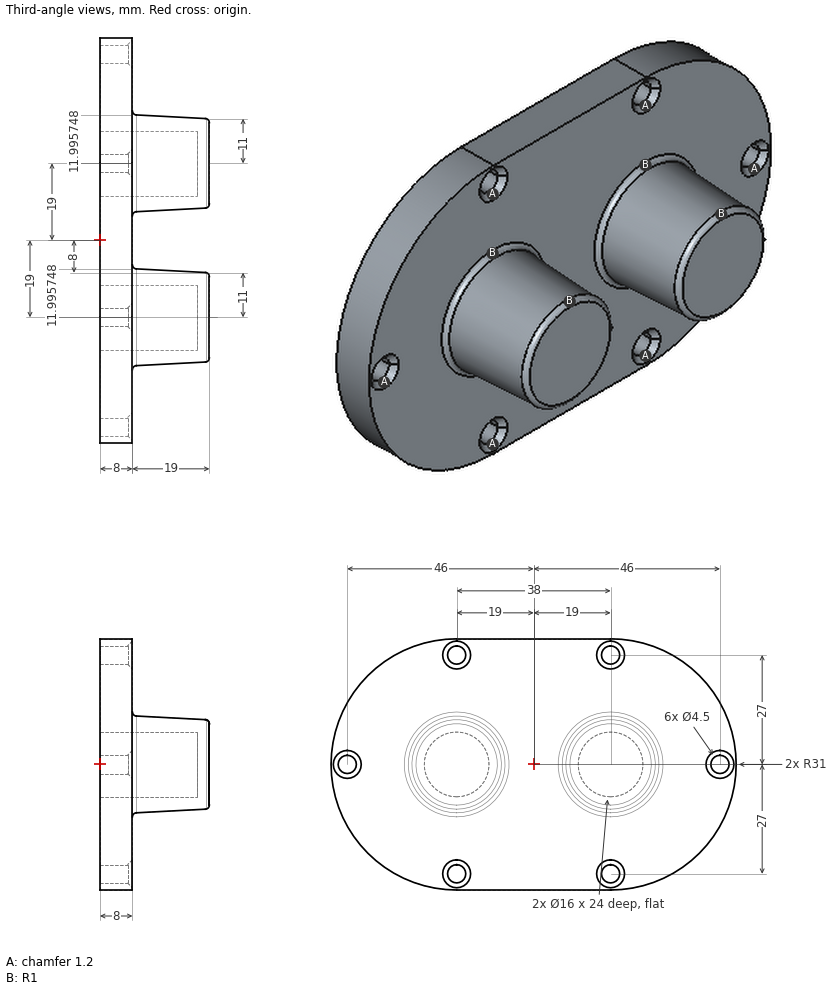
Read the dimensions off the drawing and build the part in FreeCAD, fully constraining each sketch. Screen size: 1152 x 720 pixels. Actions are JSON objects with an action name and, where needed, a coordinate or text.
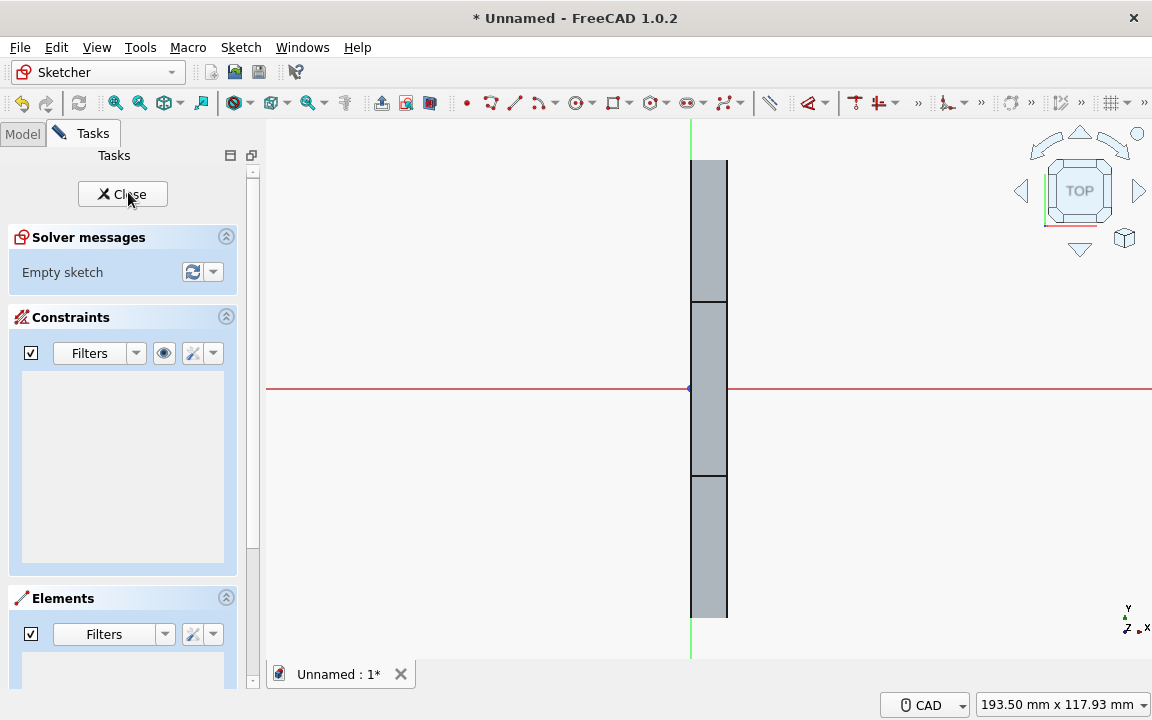
{"action": "left_click", "coordinate": [430, 104]}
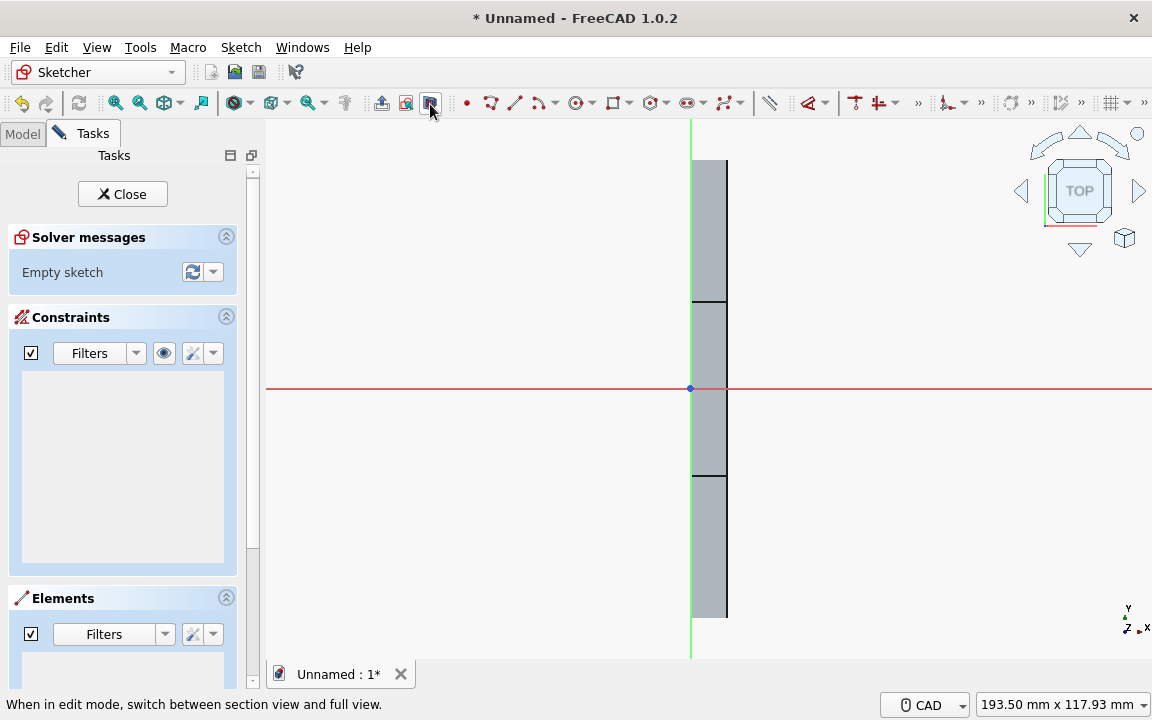
{"action": "scroll", "coordinate": [826, 451], "scroll_direction": "up", "scroll_amount": 6}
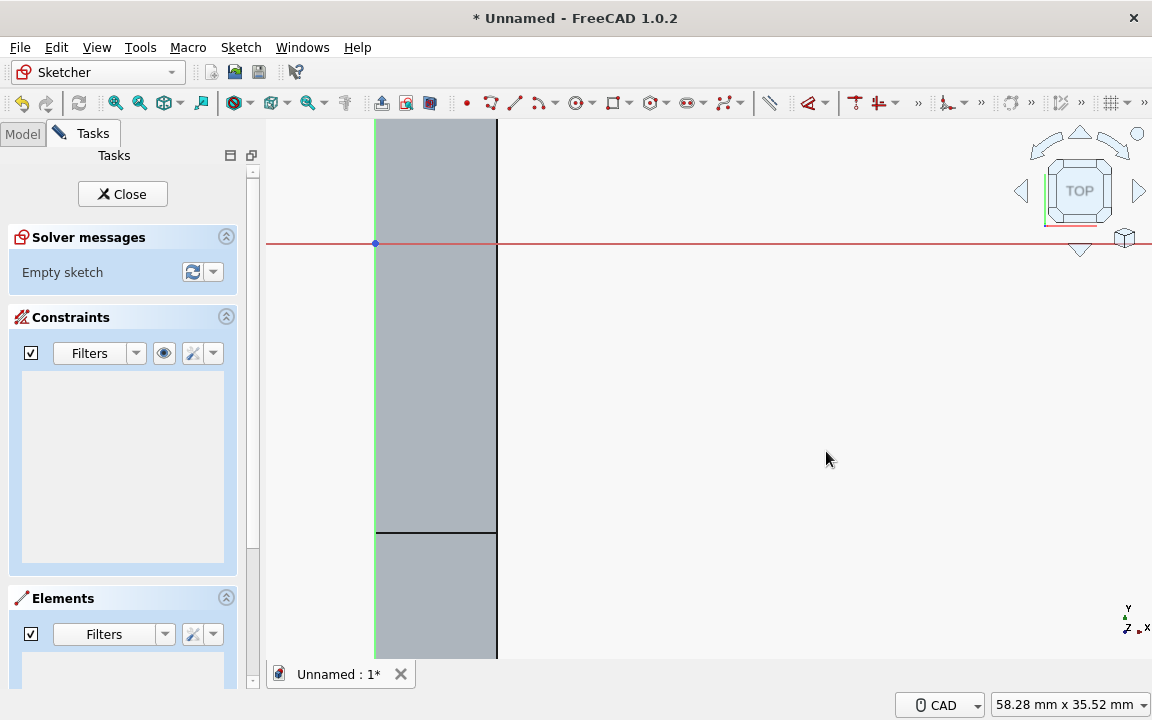
{"action": "left_click", "coordinate": [492, 104]}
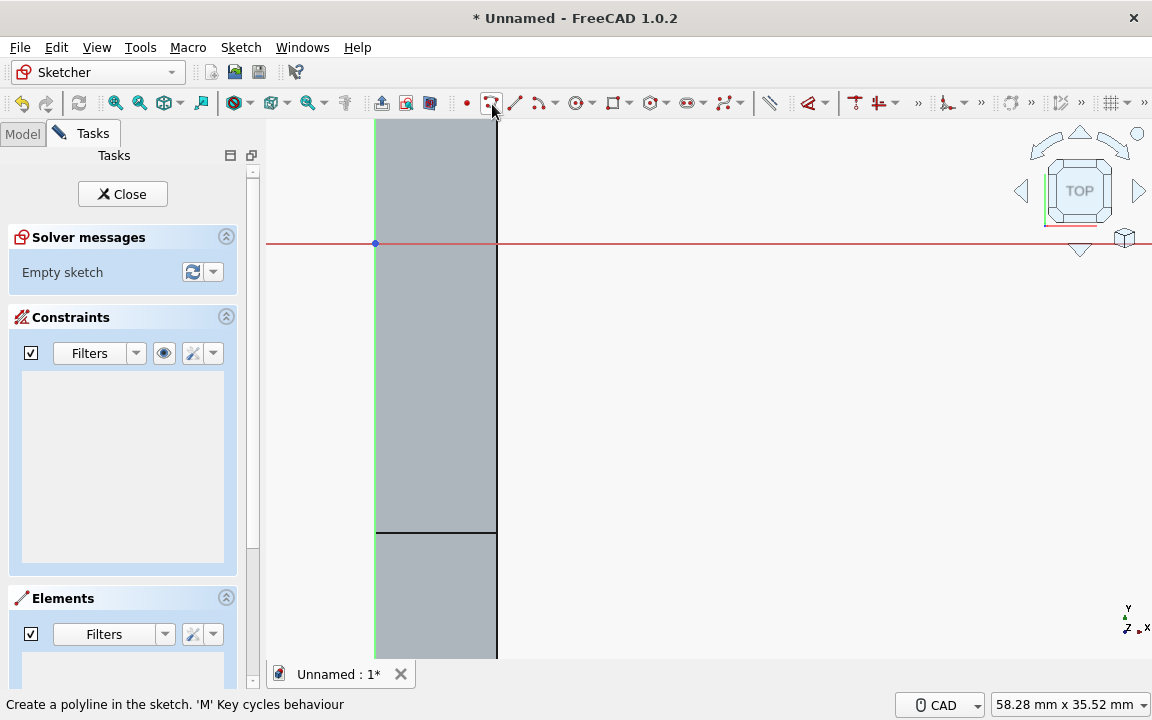
{"action": "left_click", "coordinate": [497, 350]}
{"action": "left_click", "coordinate": [497, 533]}
{"action": "left_click", "coordinate": [786, 533]}
{"action": "left_click", "coordinate": [786, 365]}
{"action": "left_click", "coordinate": [497, 351]}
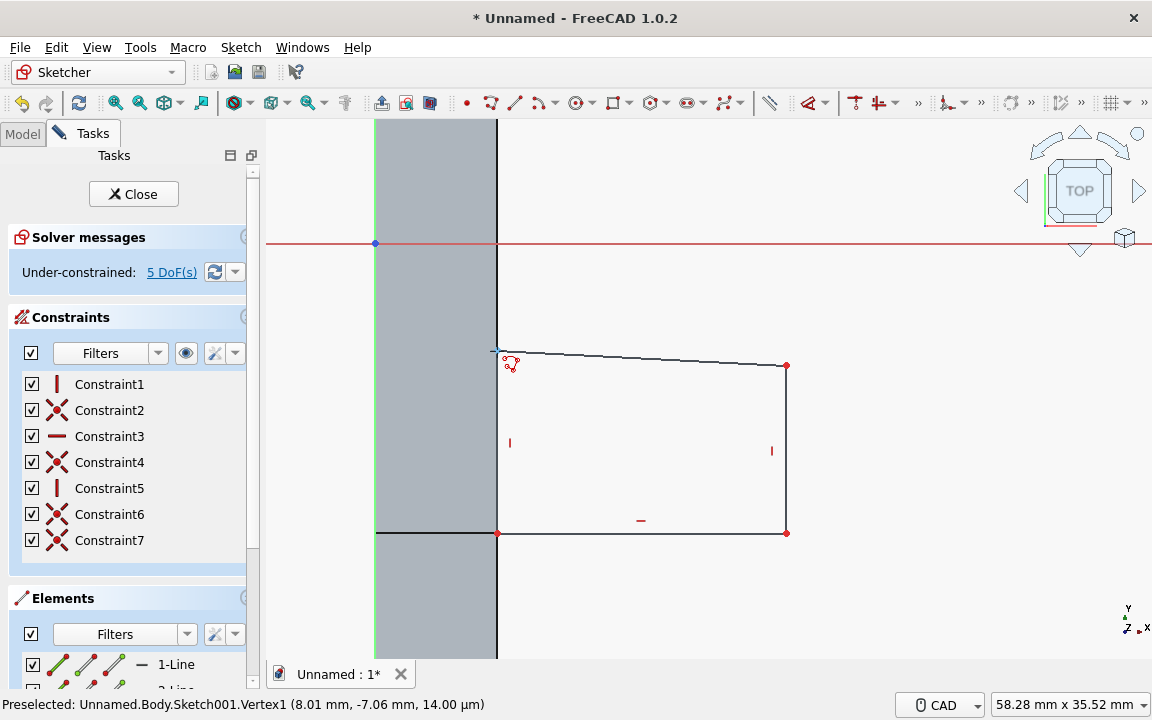
{"action": "left_click", "coordinate": [516, 104]}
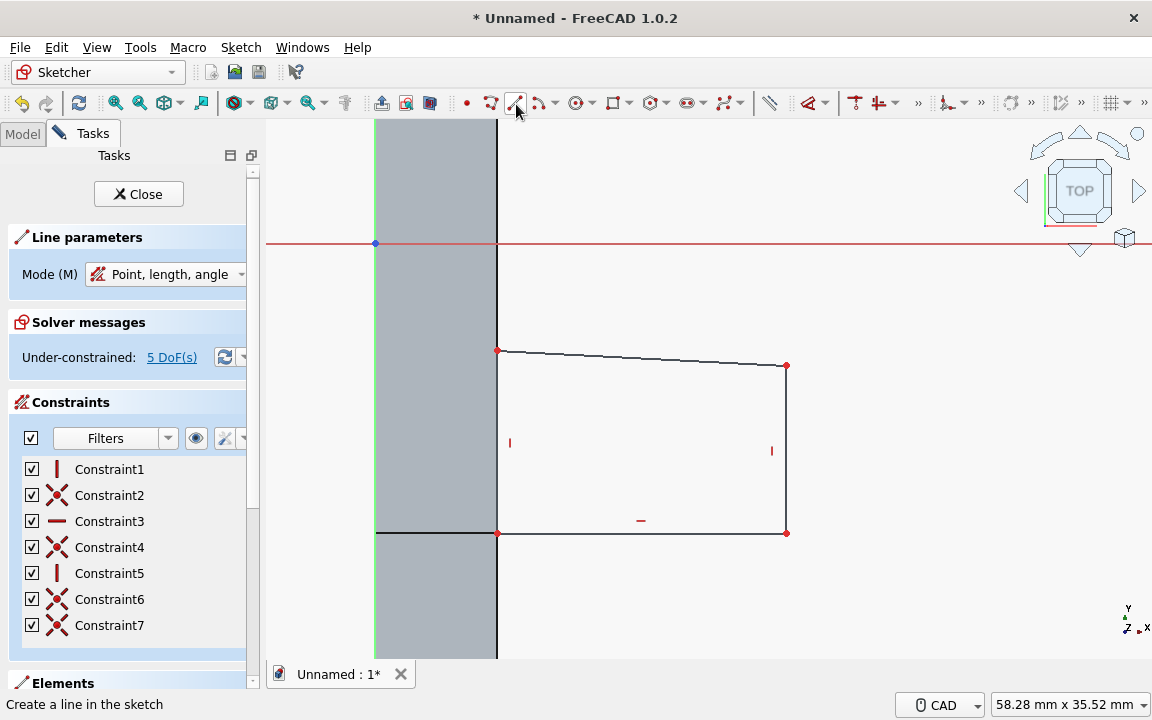
{"action": "left_click", "coordinate": [815, 533]}
{"action": "left_click", "coordinate": [901, 533]}
{"action": "key", "text": "Escape"}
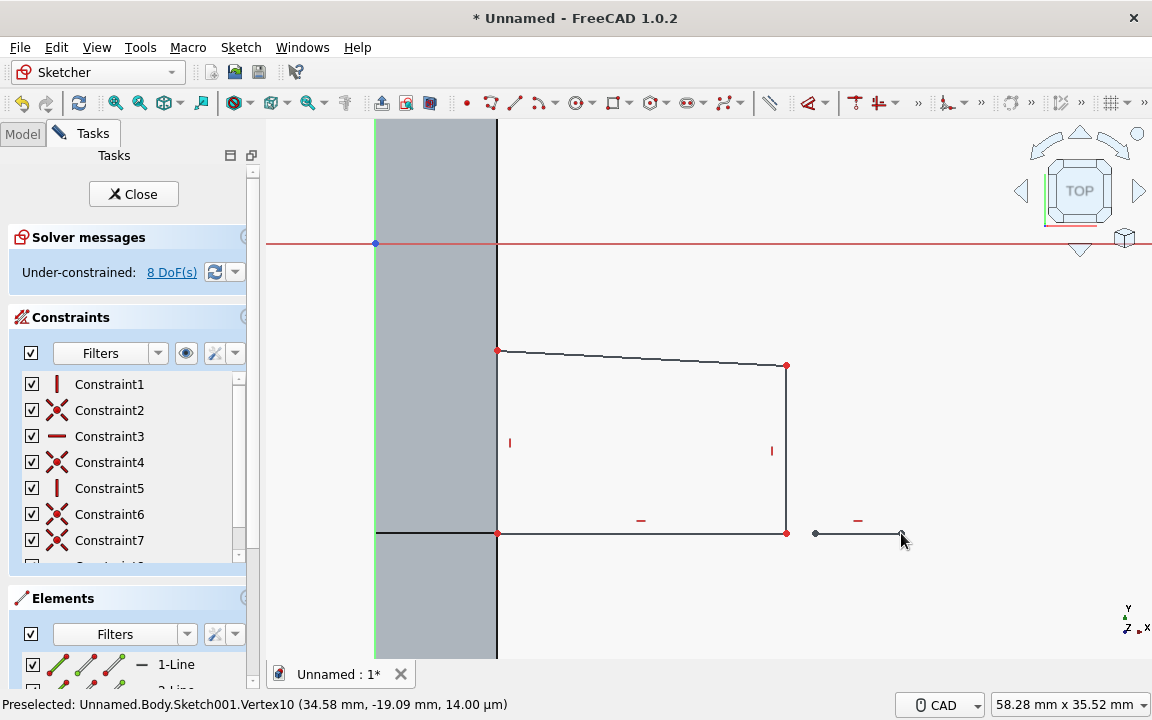
{"action": "left_click", "coordinate": [841, 534]}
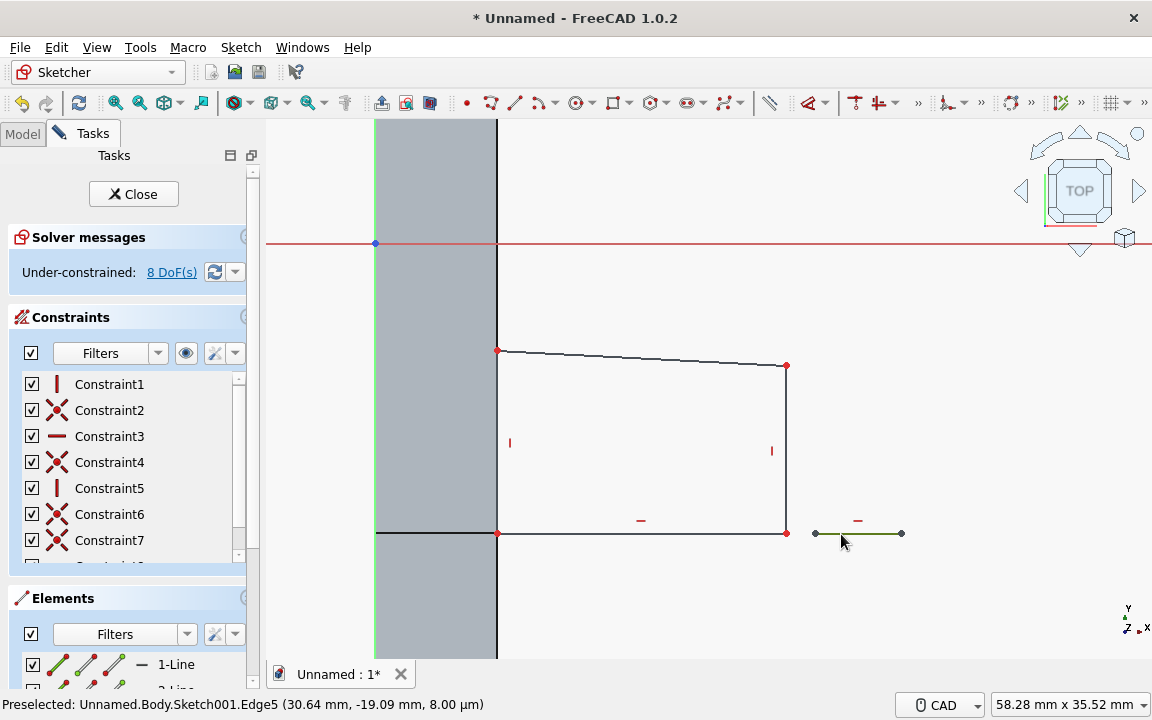
{"action": "left_click", "coordinate": [770, 104]}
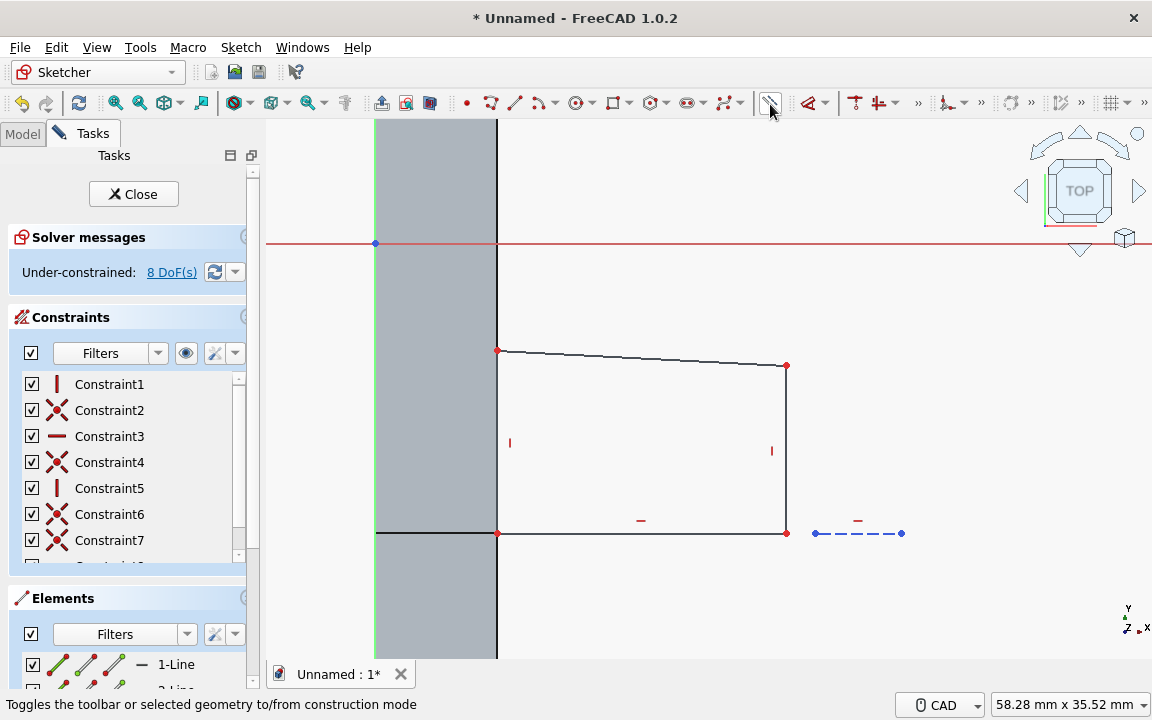
{"action": "left_click", "coordinate": [808, 104]}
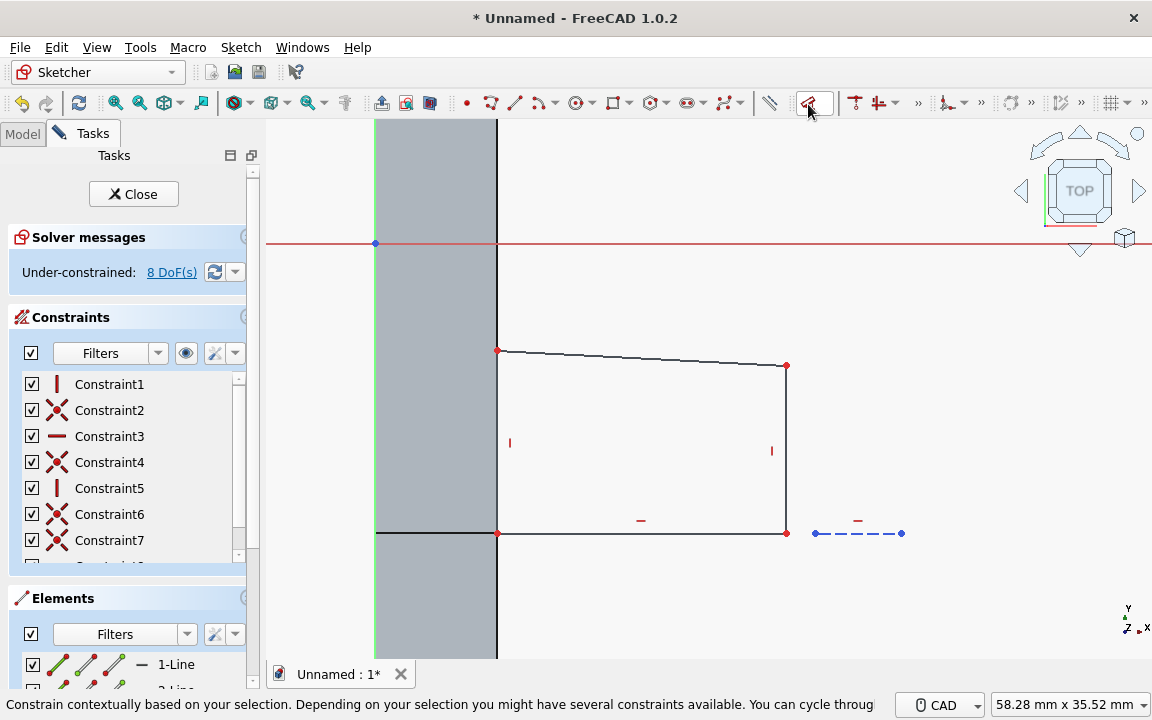
{"action": "left_click", "coordinate": [584, 534]}
{"action": "left_click", "coordinate": [641, 568]}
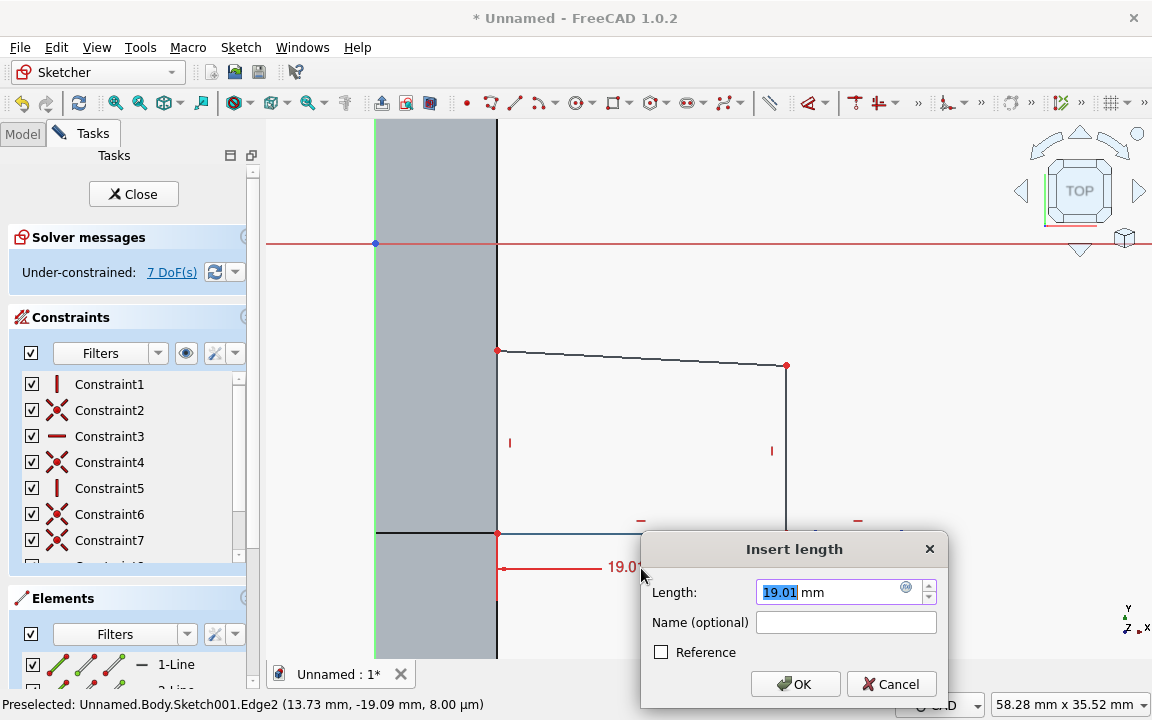
{"action": "type", "text": "19"}
{"action": "key", "text": "Return"}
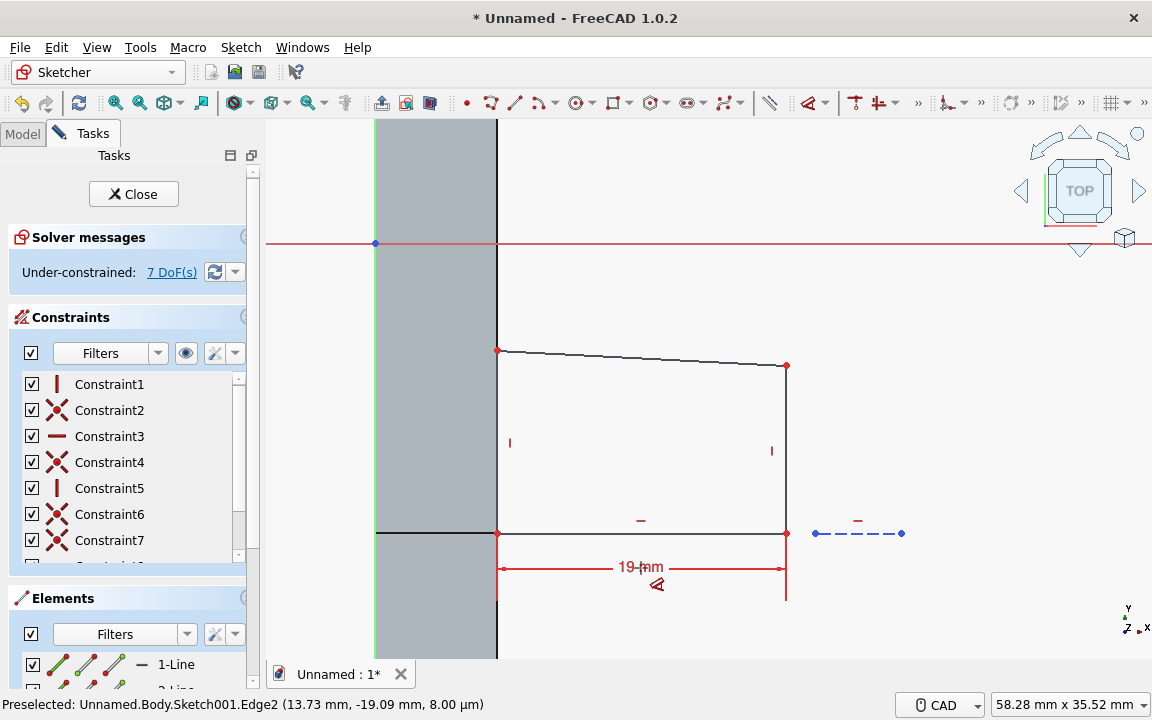
{"action": "left_click", "coordinate": [786, 484]}
{"action": "left_click", "coordinate": [820, 450]}